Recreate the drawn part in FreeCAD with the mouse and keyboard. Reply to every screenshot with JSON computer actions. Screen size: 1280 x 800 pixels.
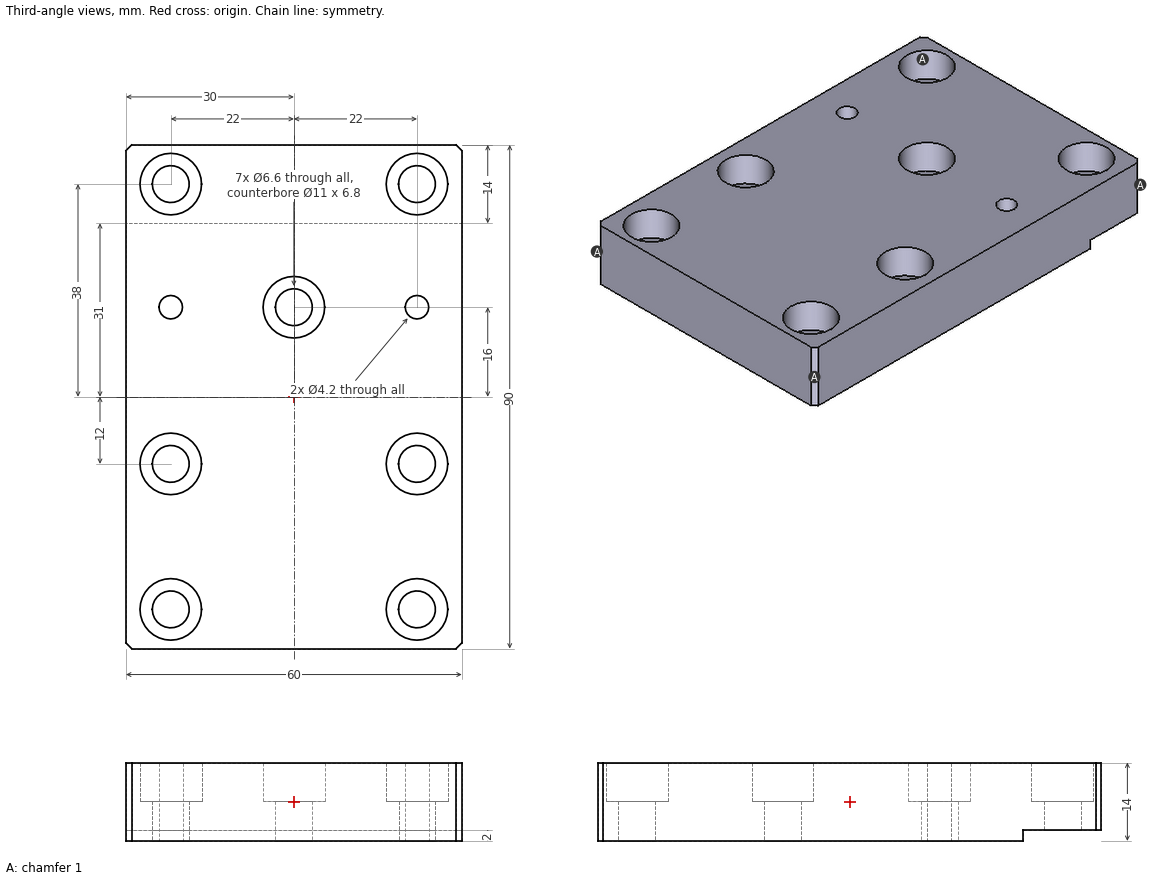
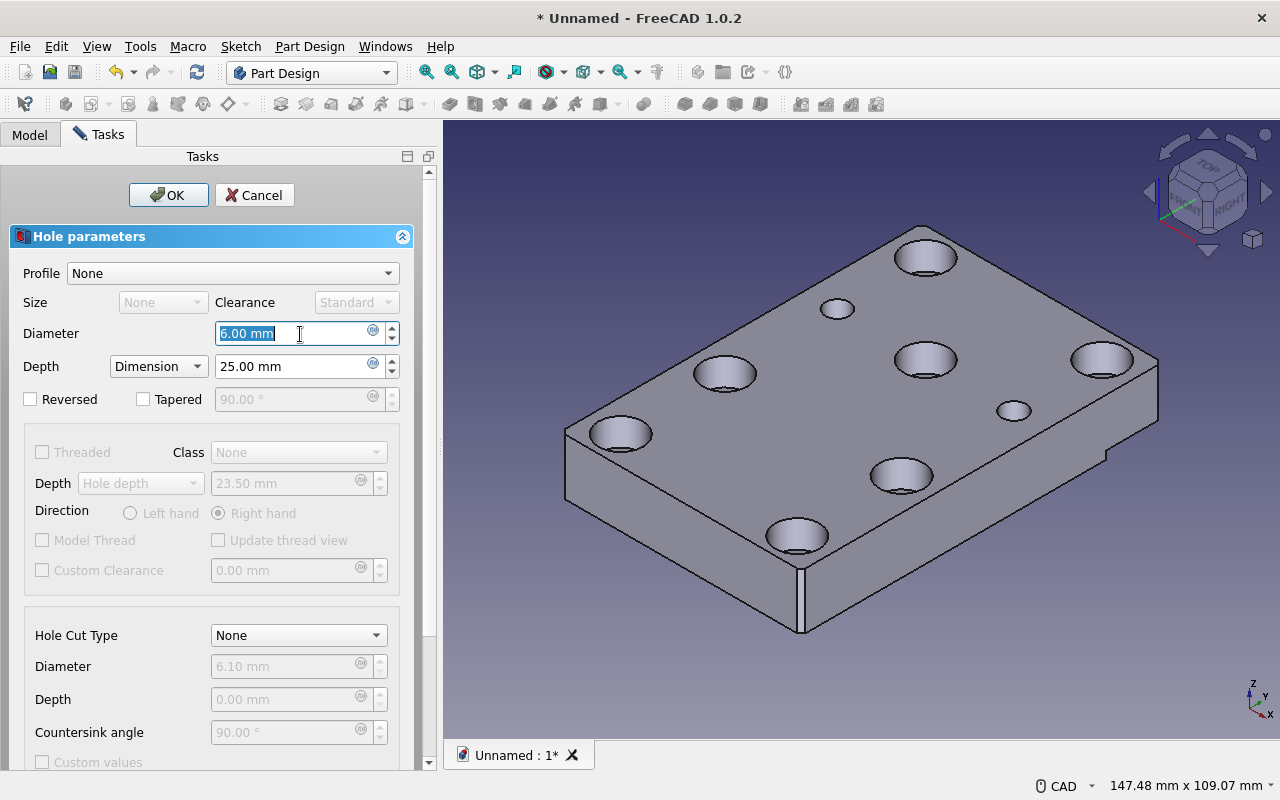
{"action": "type", "text": "4.2"}
{"action": "key", "text": "Tab"}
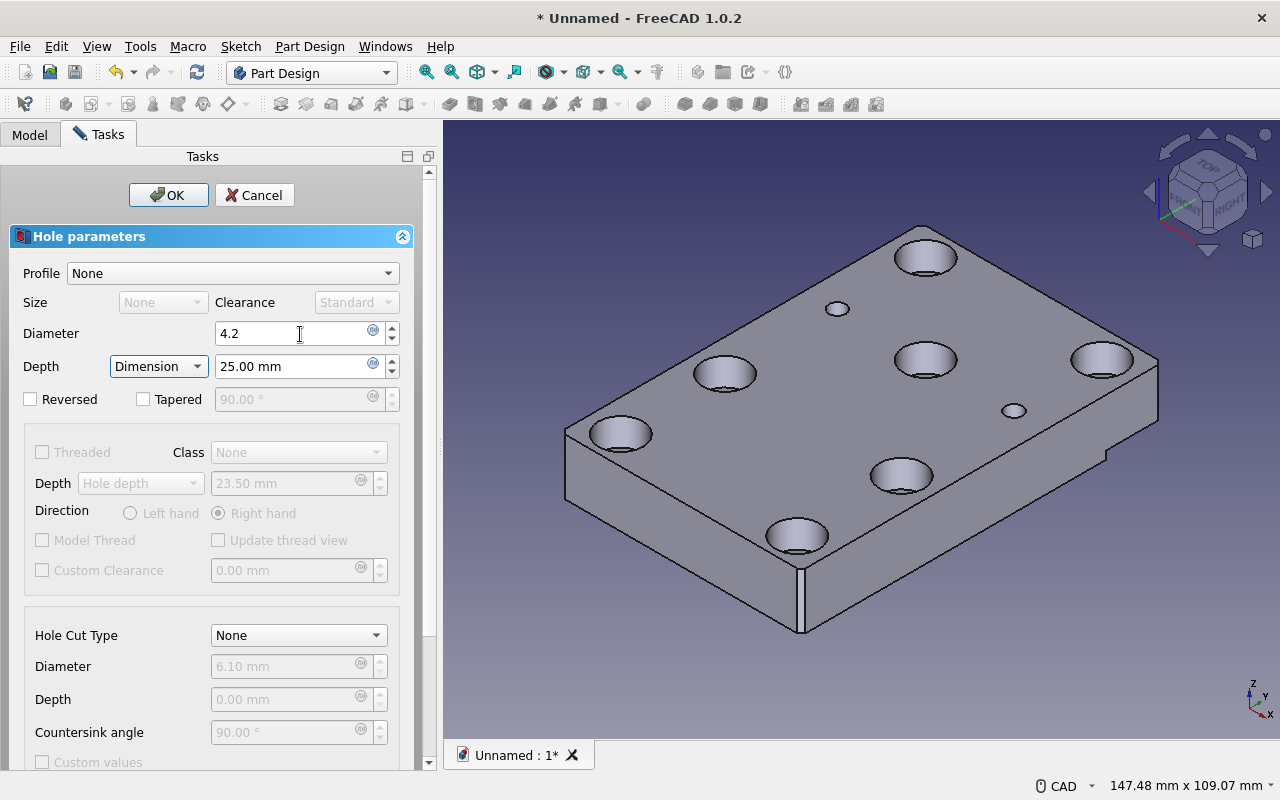
{"action": "left_click", "coordinate": [160, 366]}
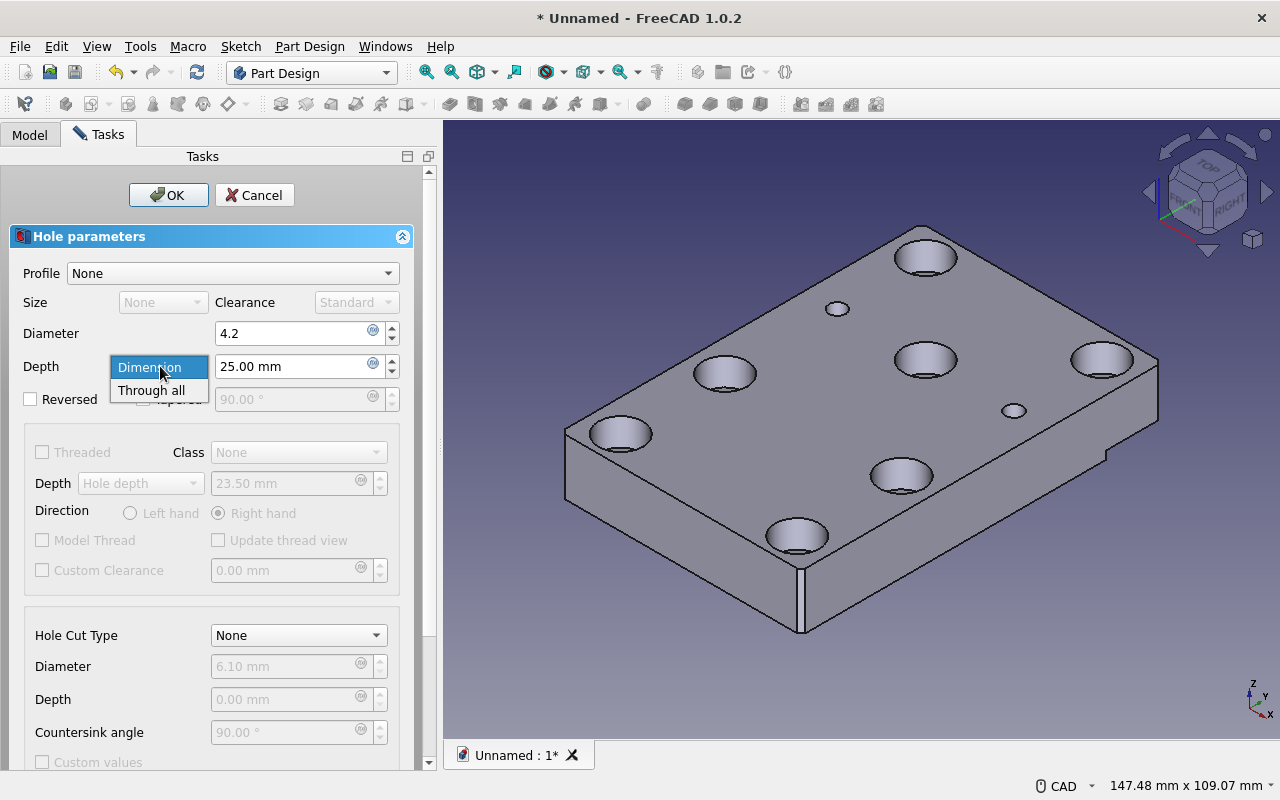
{"action": "left_click", "coordinate": [158, 390]}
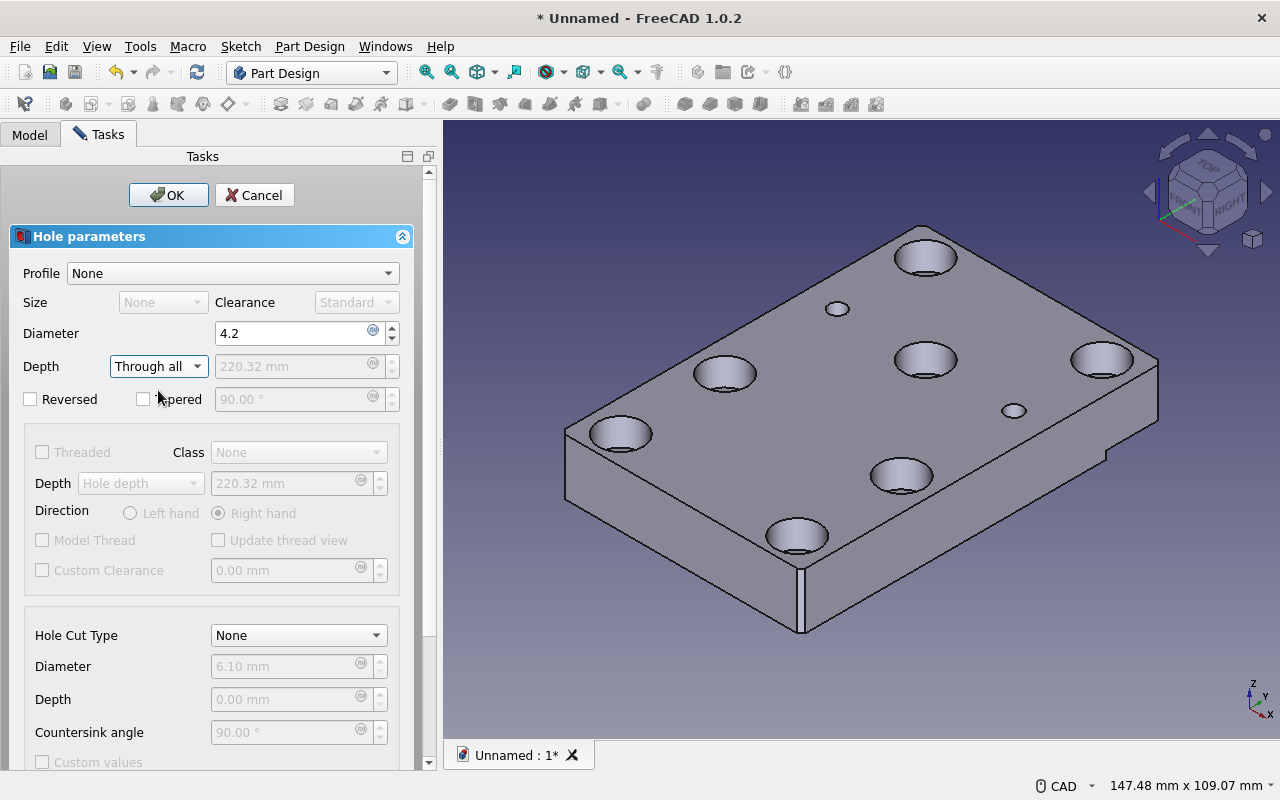
{"action": "left_click", "coordinate": [169, 195]}